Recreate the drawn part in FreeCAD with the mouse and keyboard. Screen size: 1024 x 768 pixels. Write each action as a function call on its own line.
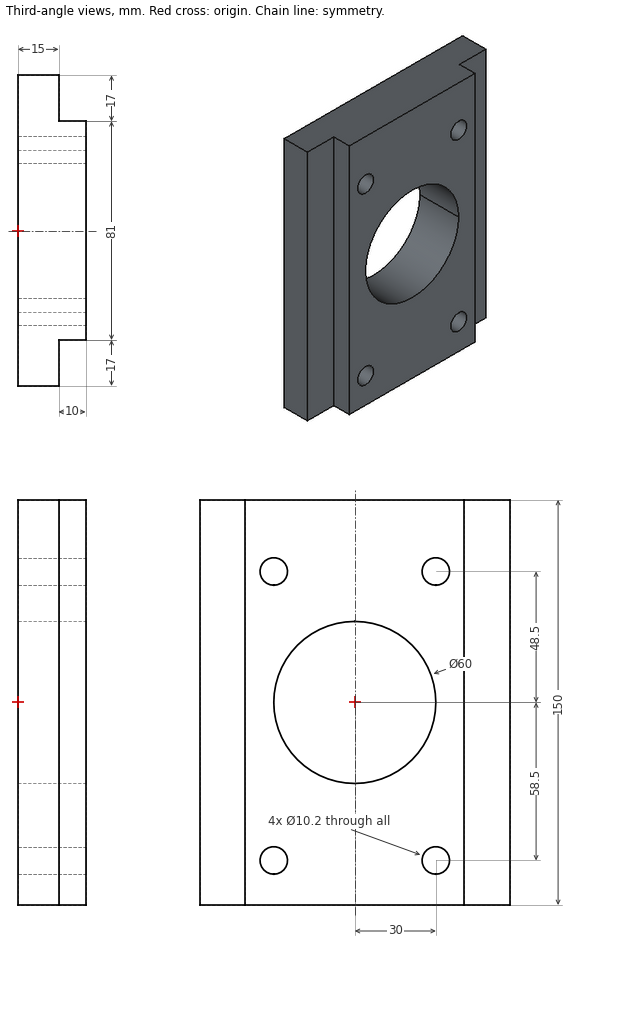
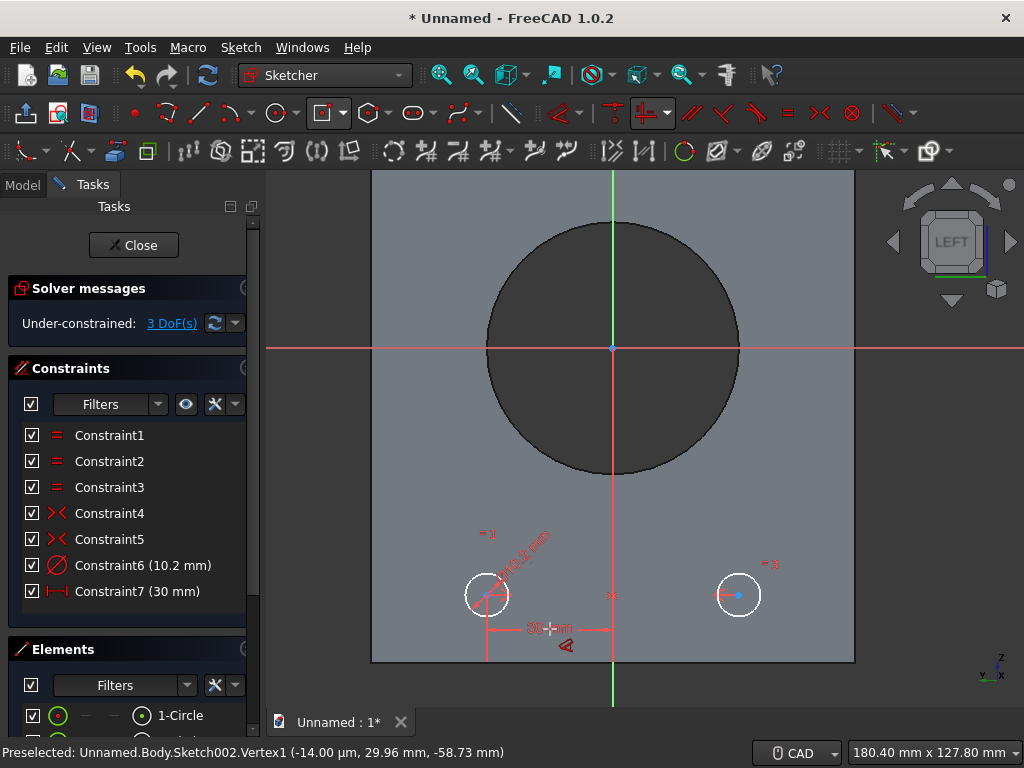
scroll(502, 579, down, 2)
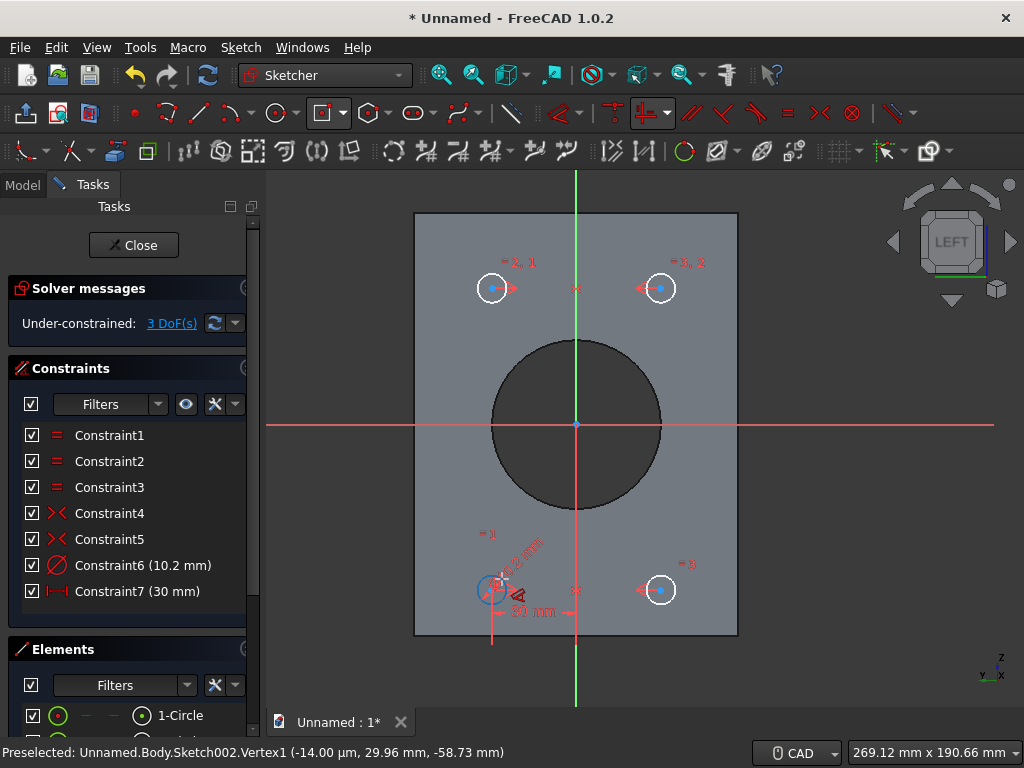
click(492, 288)
click(534, 254)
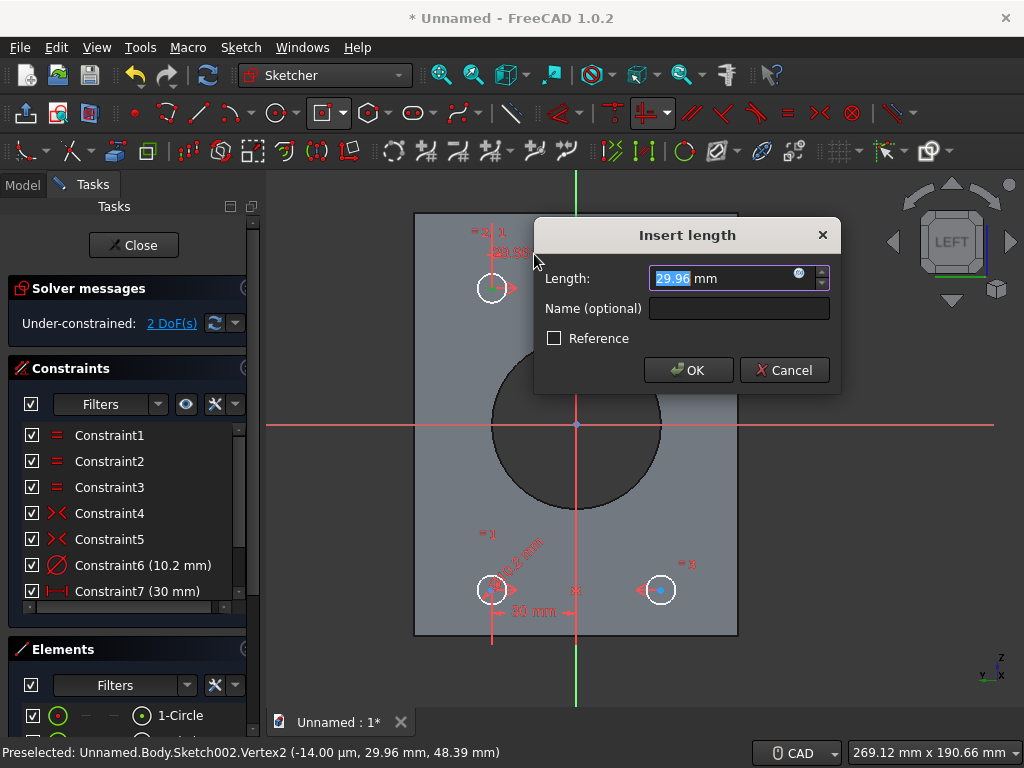
text(30)
key(Return)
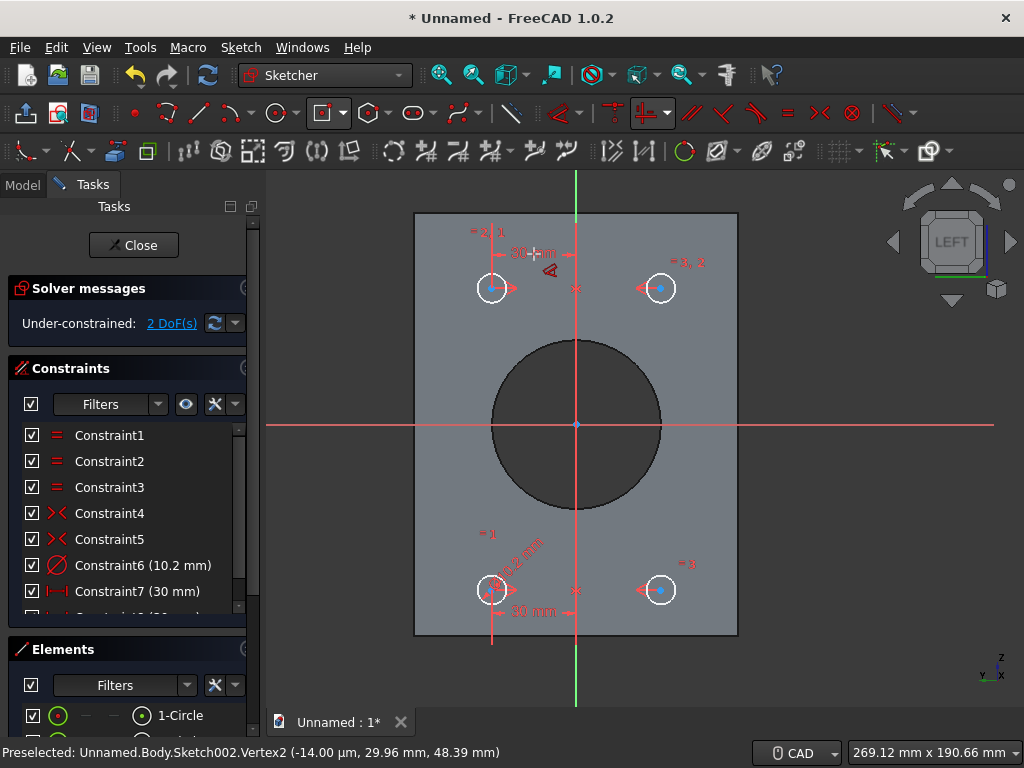
click(492, 590)
click(458, 507)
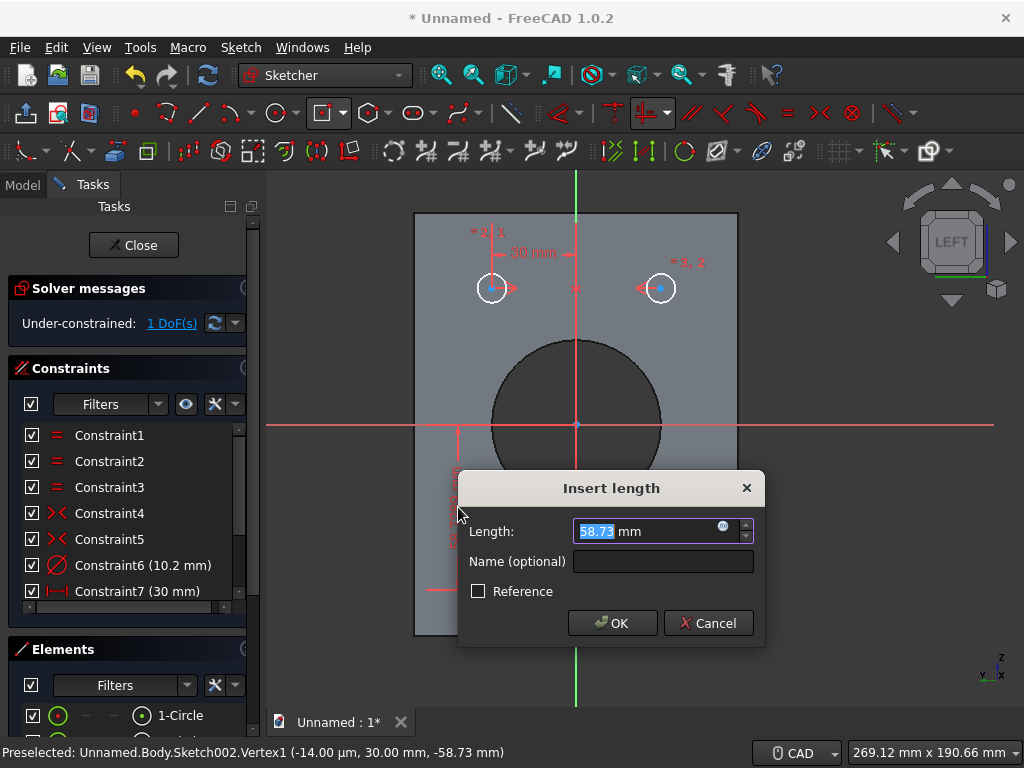
text(58.5)
key(Return)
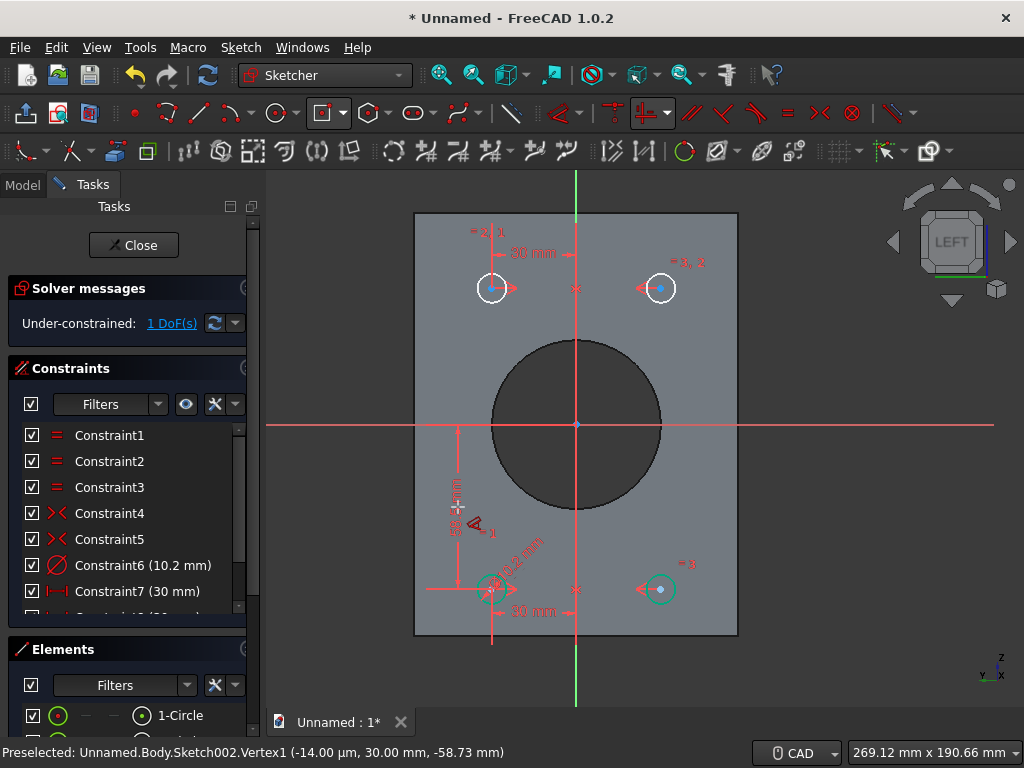
click(492, 288)
click(458, 356)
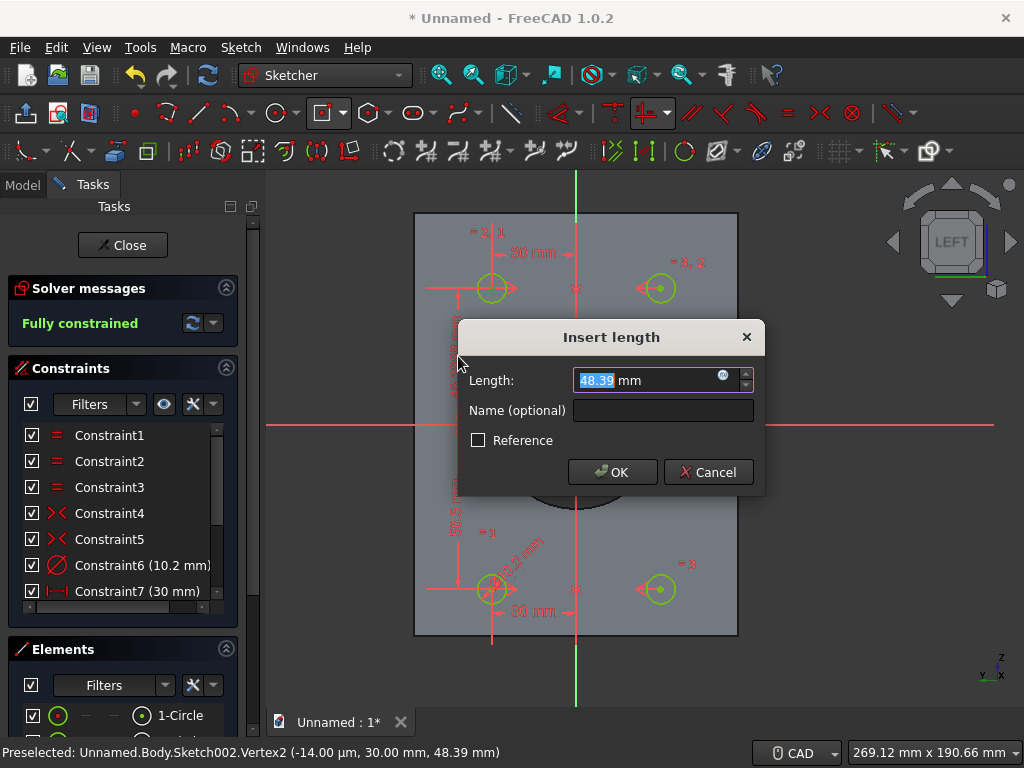
text(48.5)
key(Return)
key(Escape)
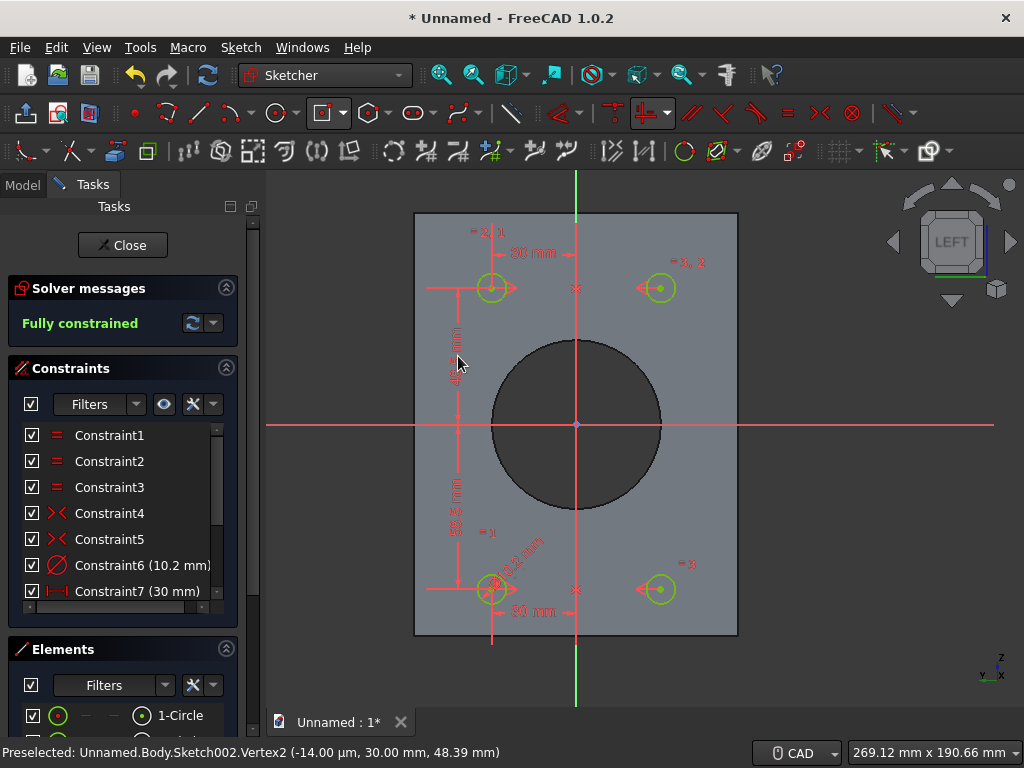
click(123, 245)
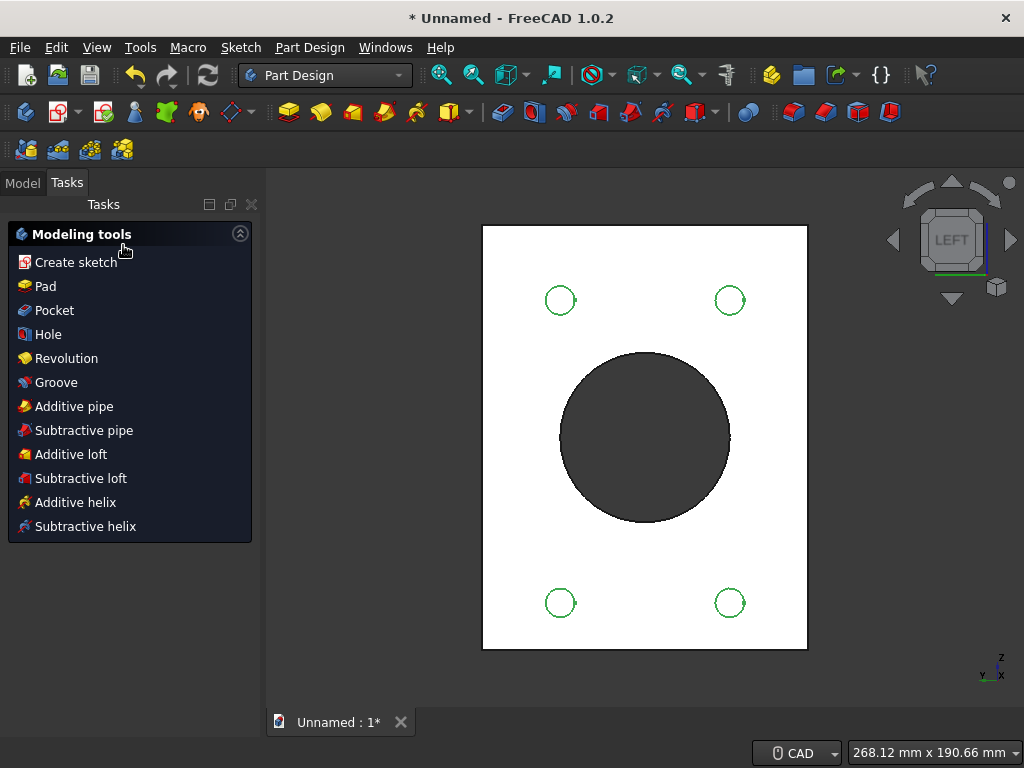
click(536, 112)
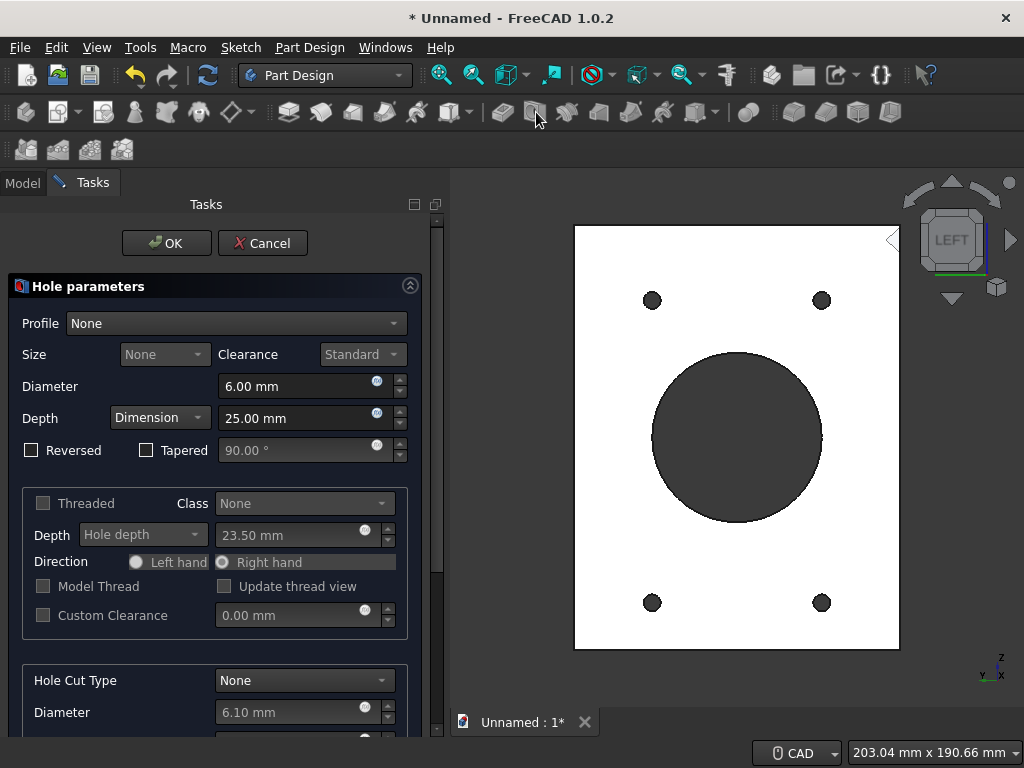
triple_click(305, 386)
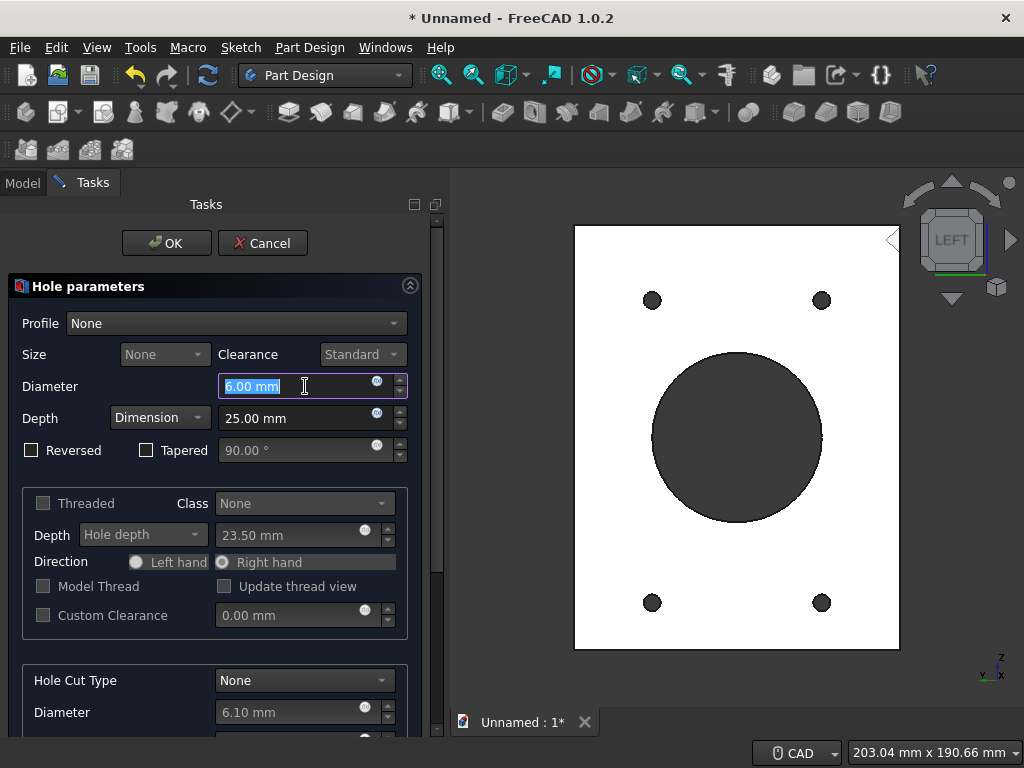
text(10.2)
key(Tab)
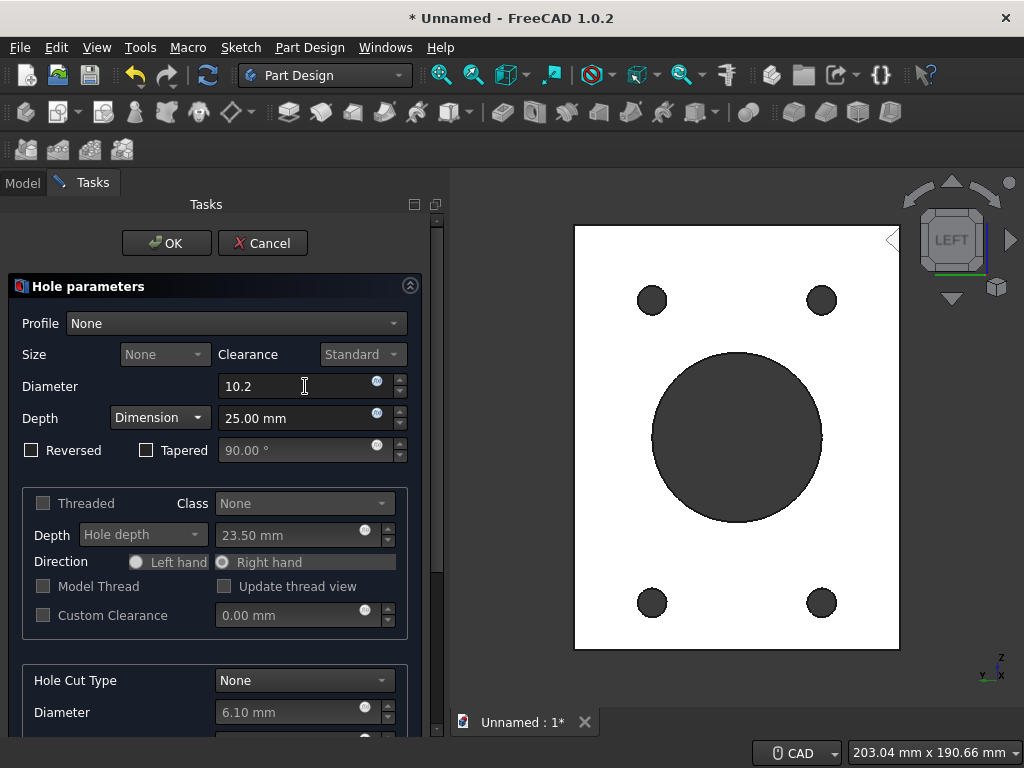
click(161, 418)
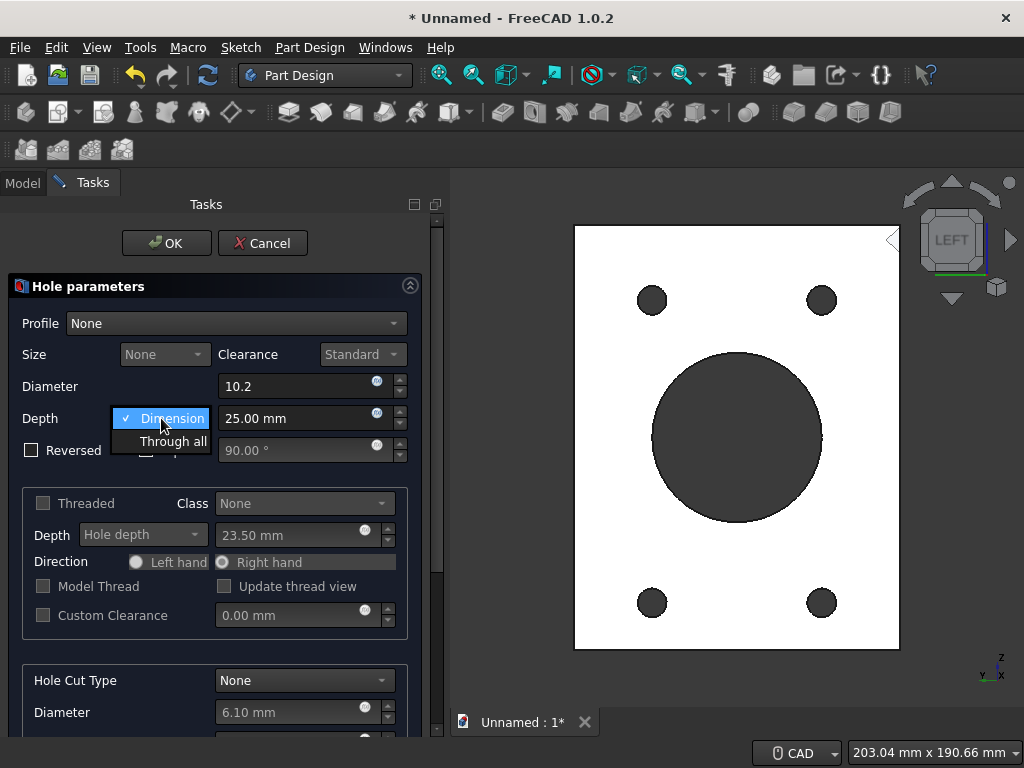
click(160, 442)